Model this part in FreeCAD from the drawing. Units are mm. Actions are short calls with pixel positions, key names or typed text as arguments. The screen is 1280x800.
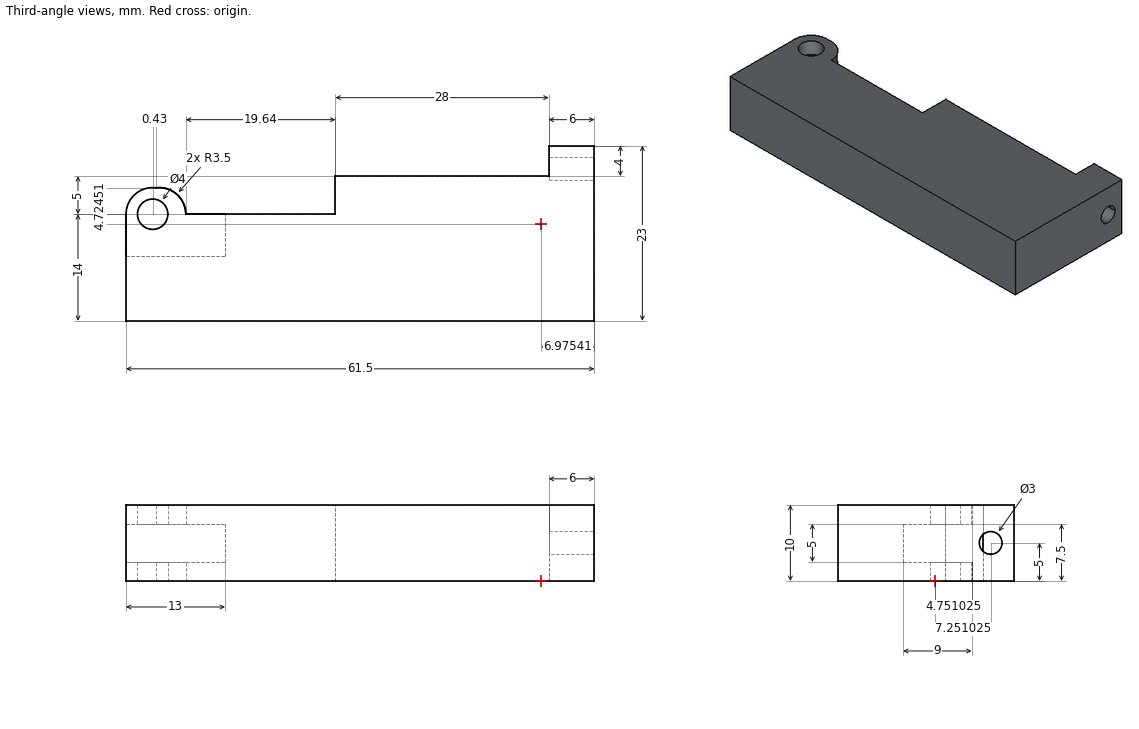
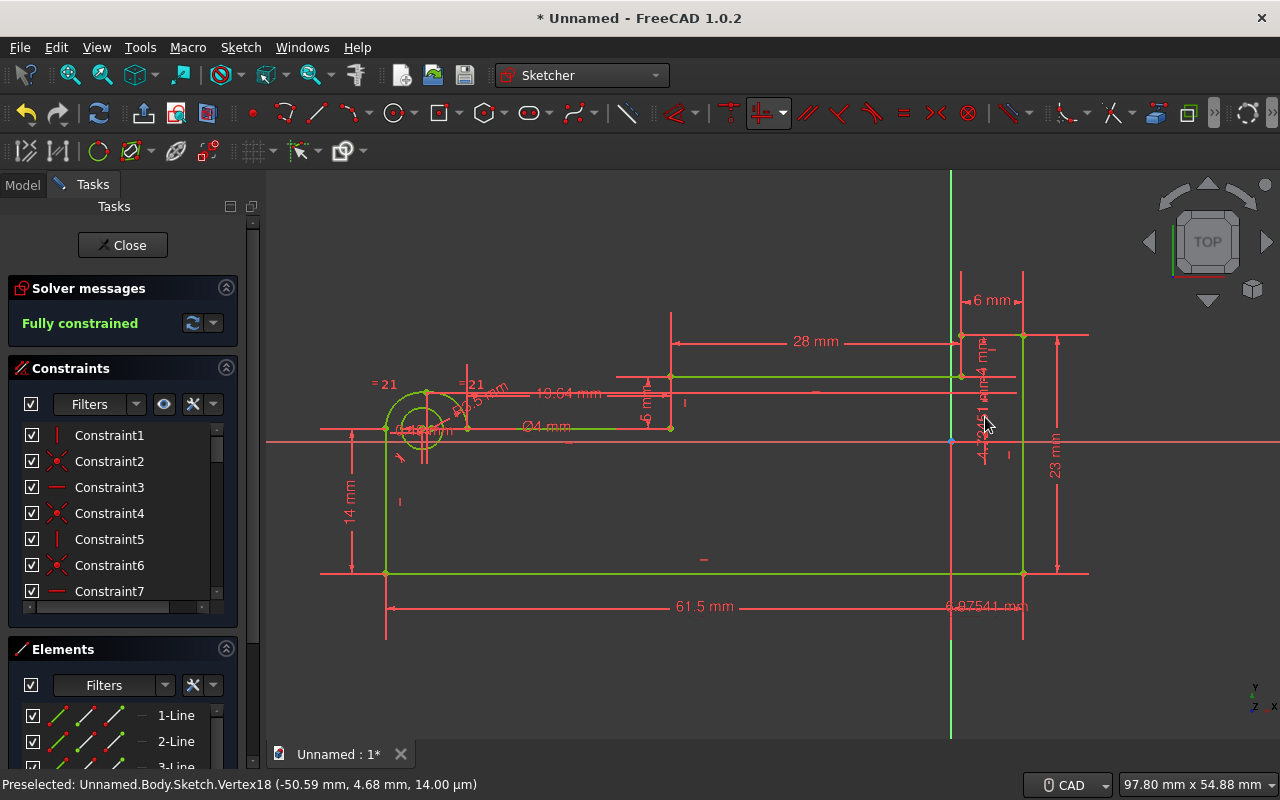
click(123, 245)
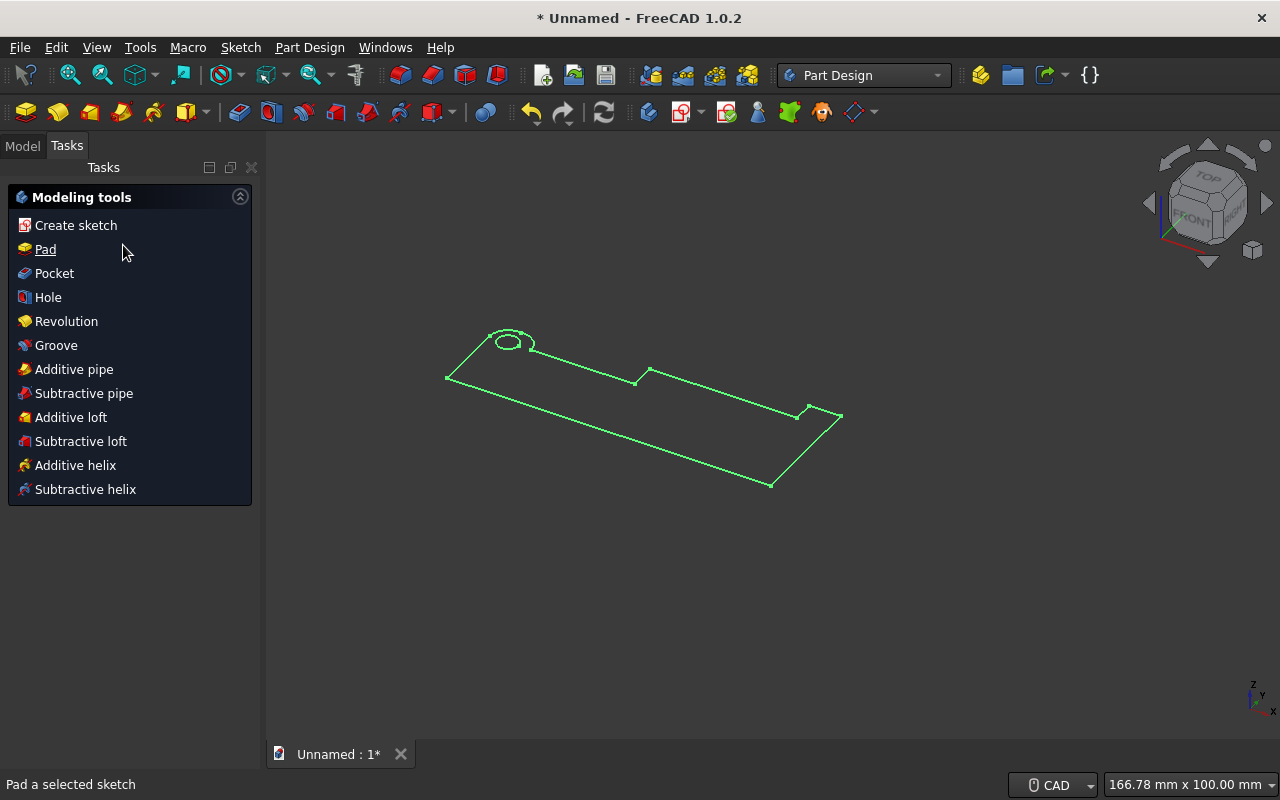
click(26, 112)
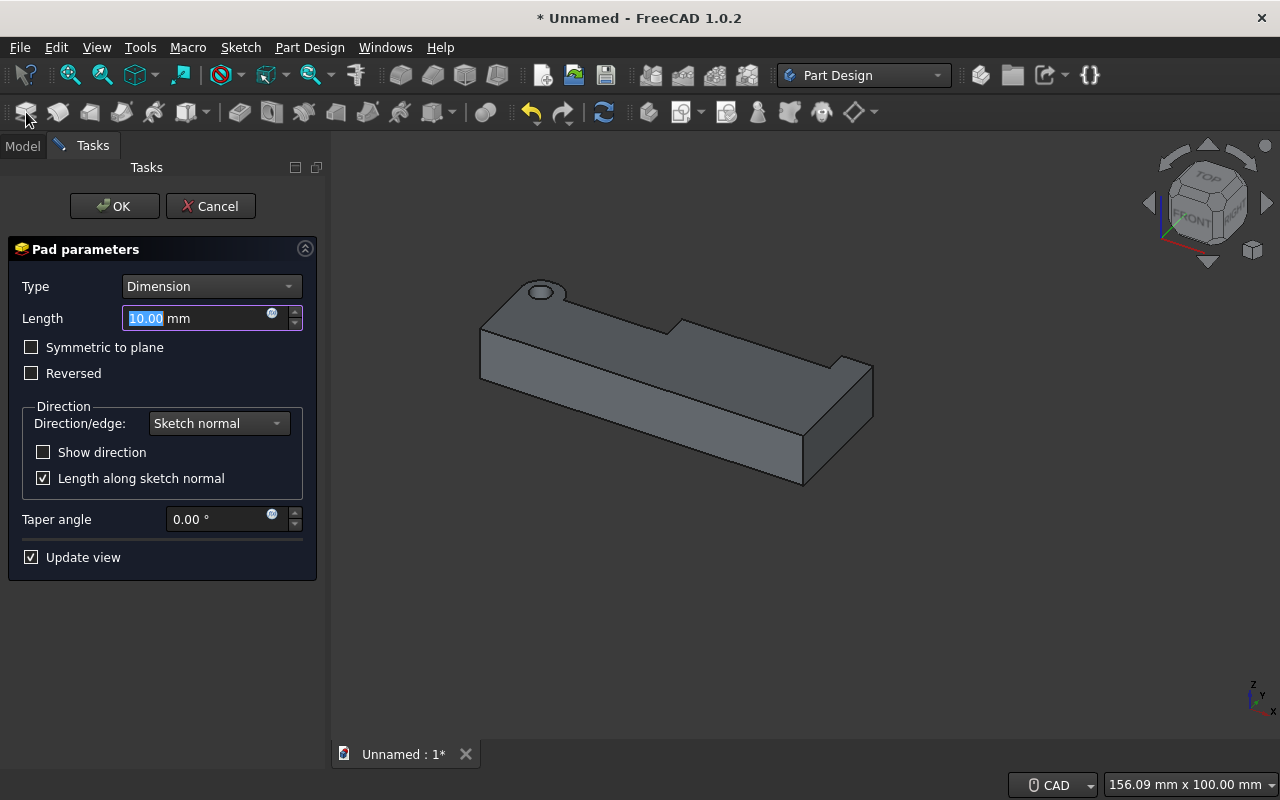
text(10)
key(Tab)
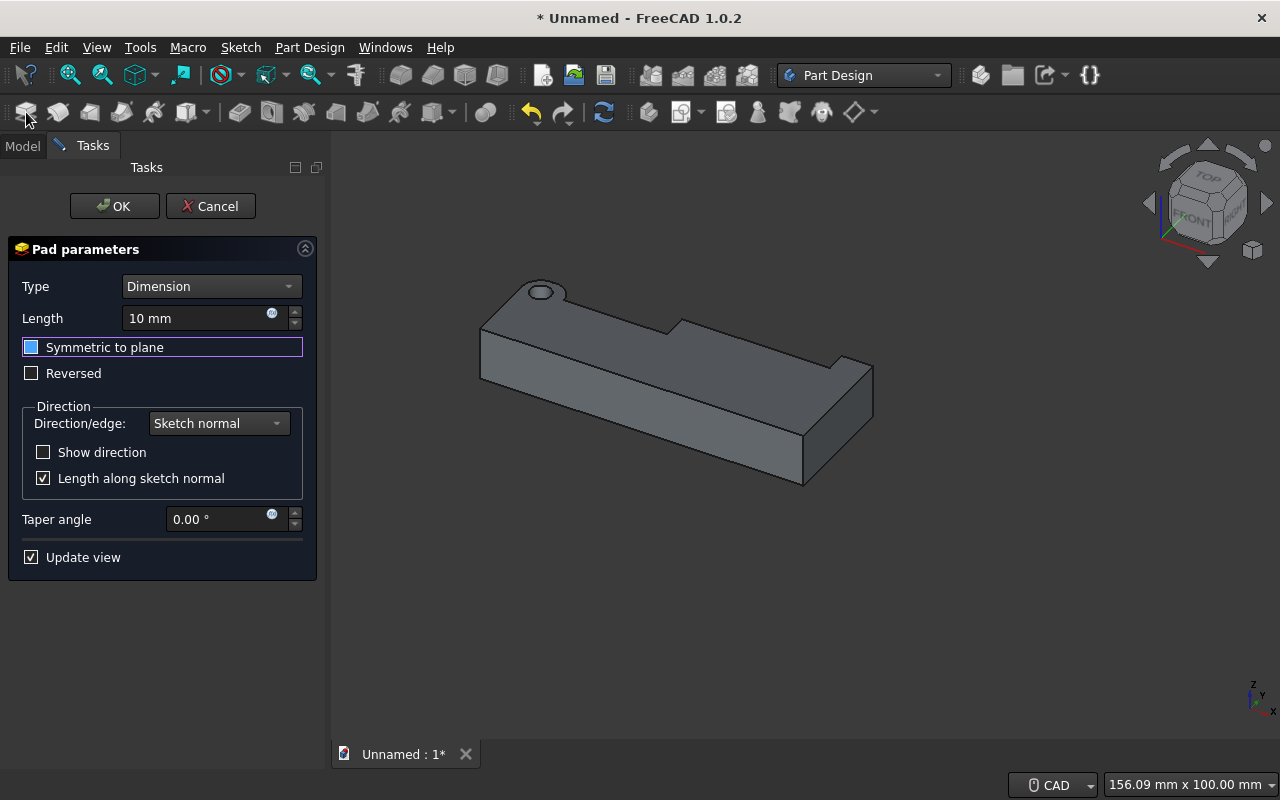
click(115, 206)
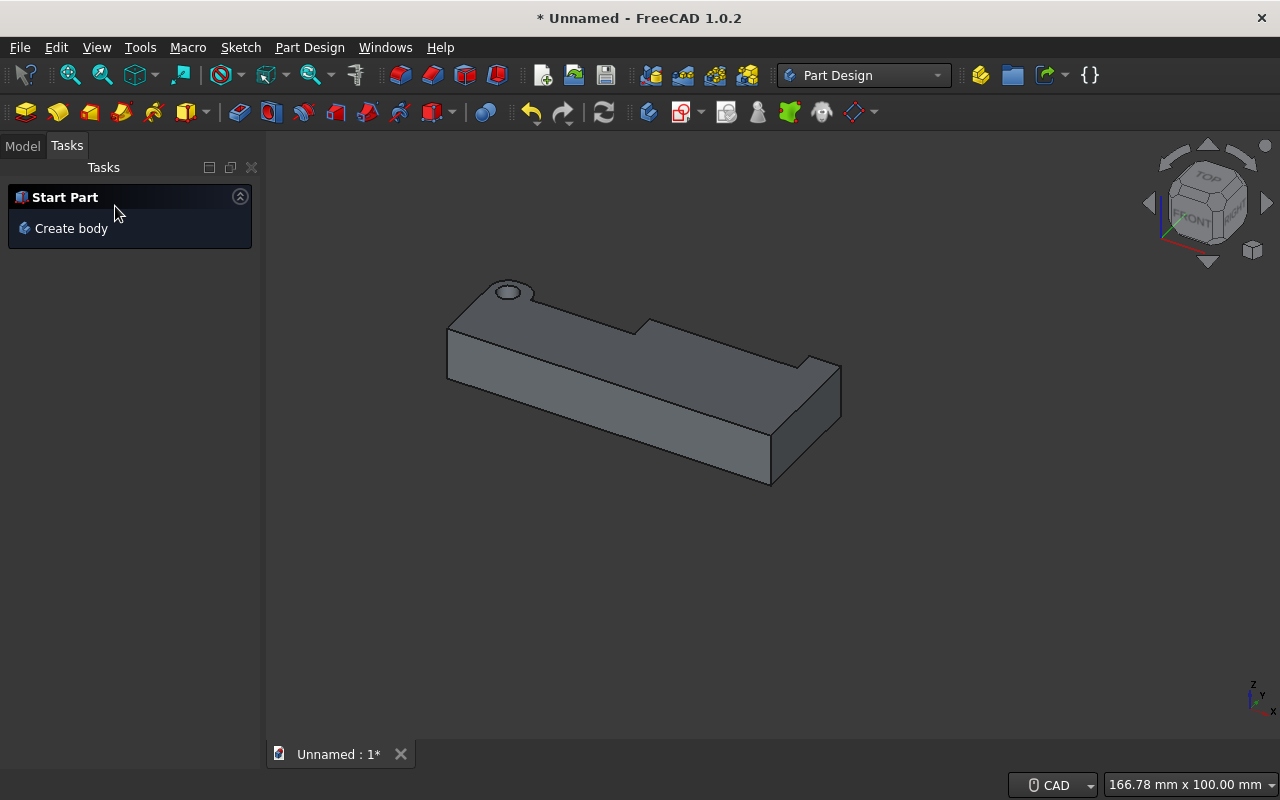
key(v)
key(f)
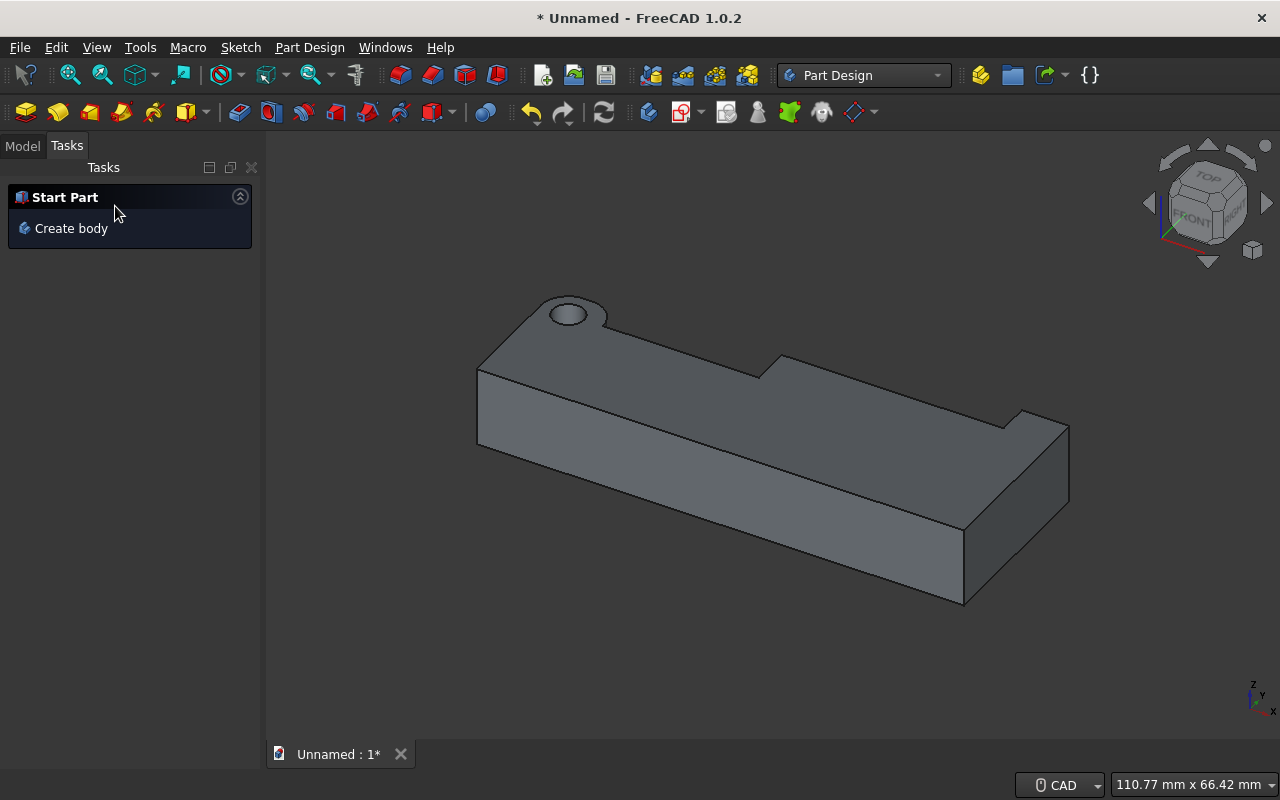
click(1032, 500)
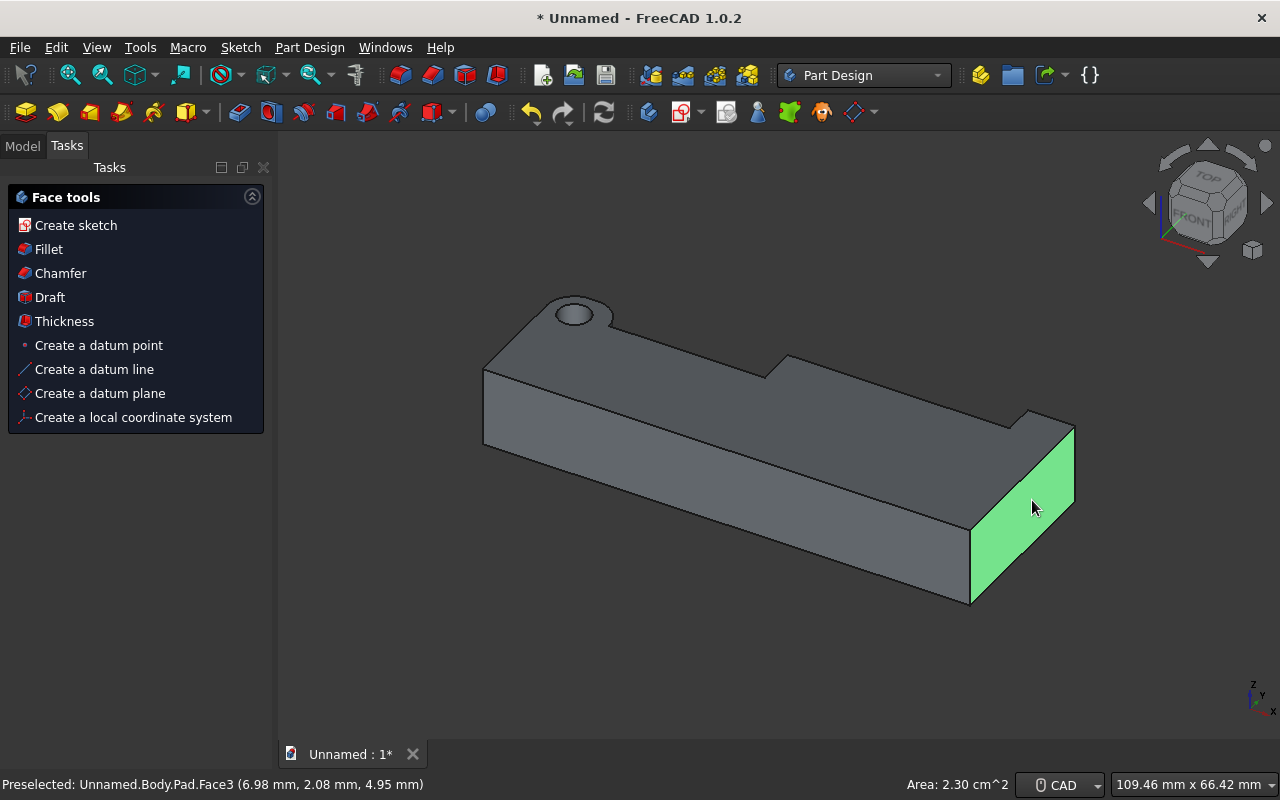
click(682, 112)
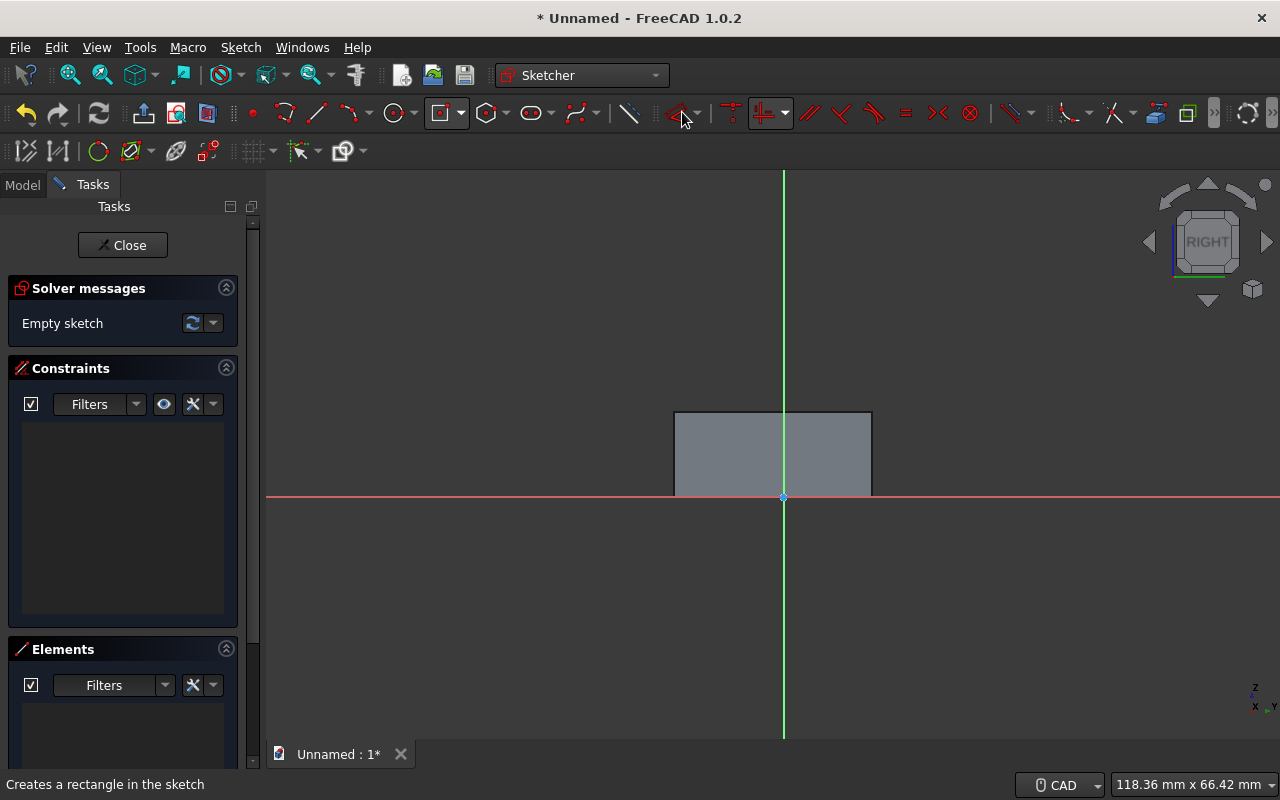
scroll(857, 454, up, 13)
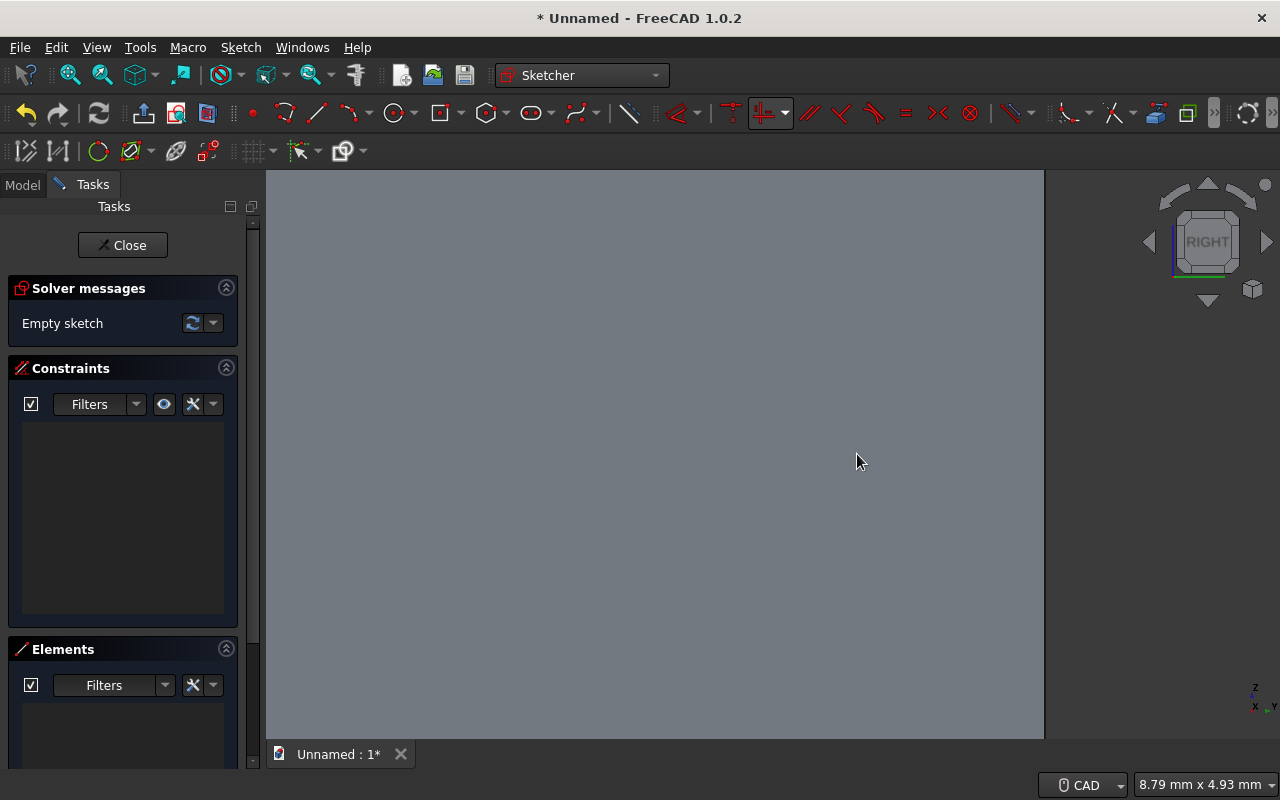
click(394, 114)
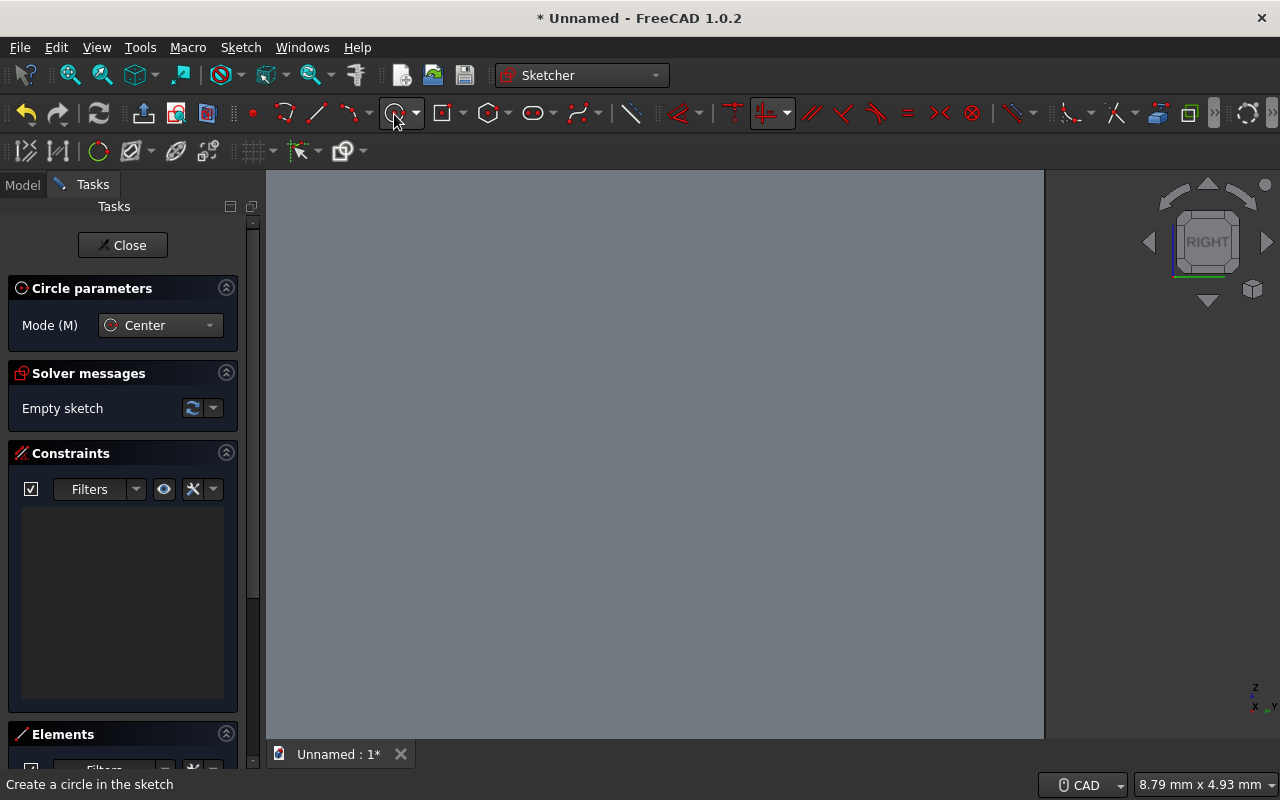
click(699, 454)
move(822, 332)